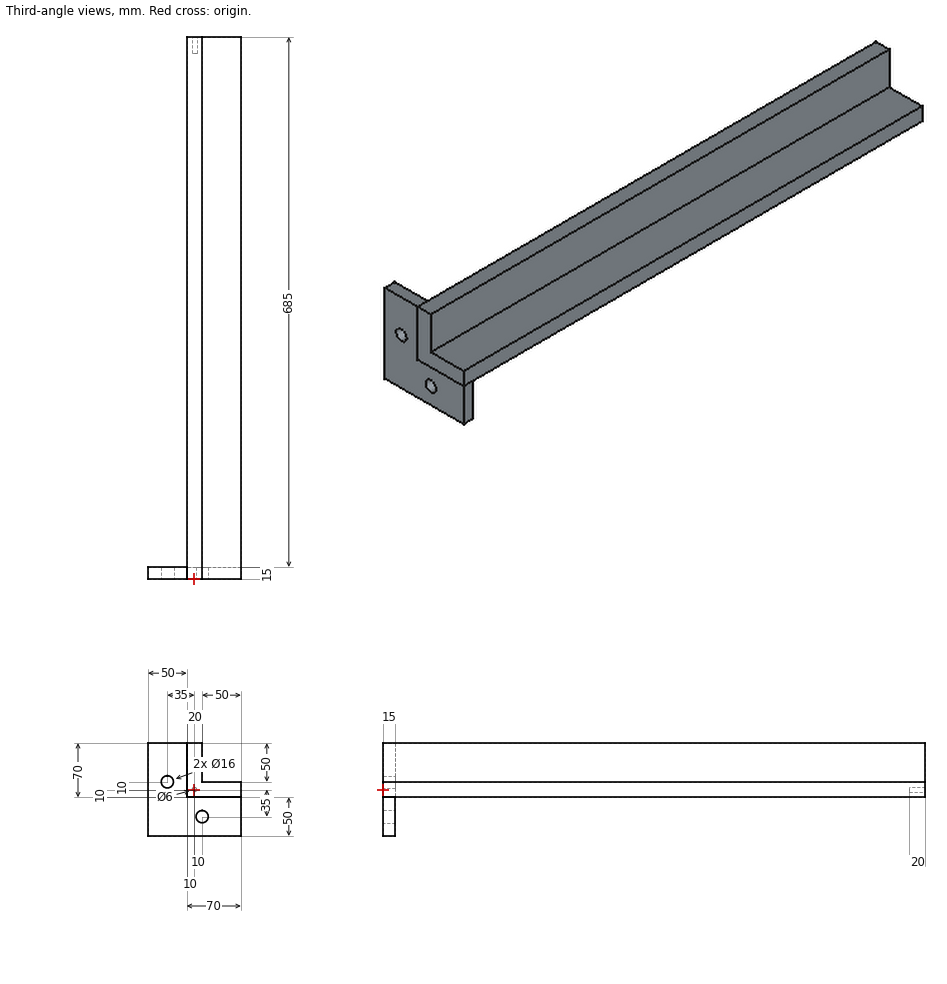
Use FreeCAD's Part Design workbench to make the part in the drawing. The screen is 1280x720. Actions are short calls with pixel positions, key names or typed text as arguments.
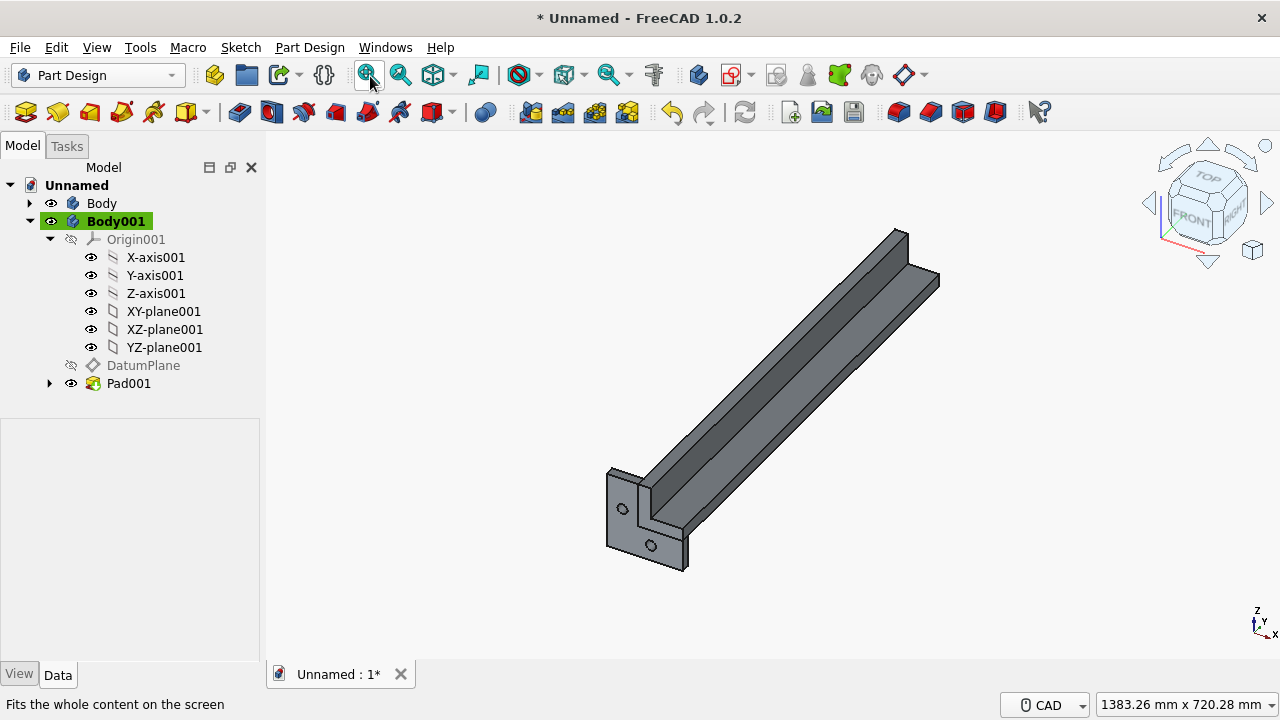
key(4)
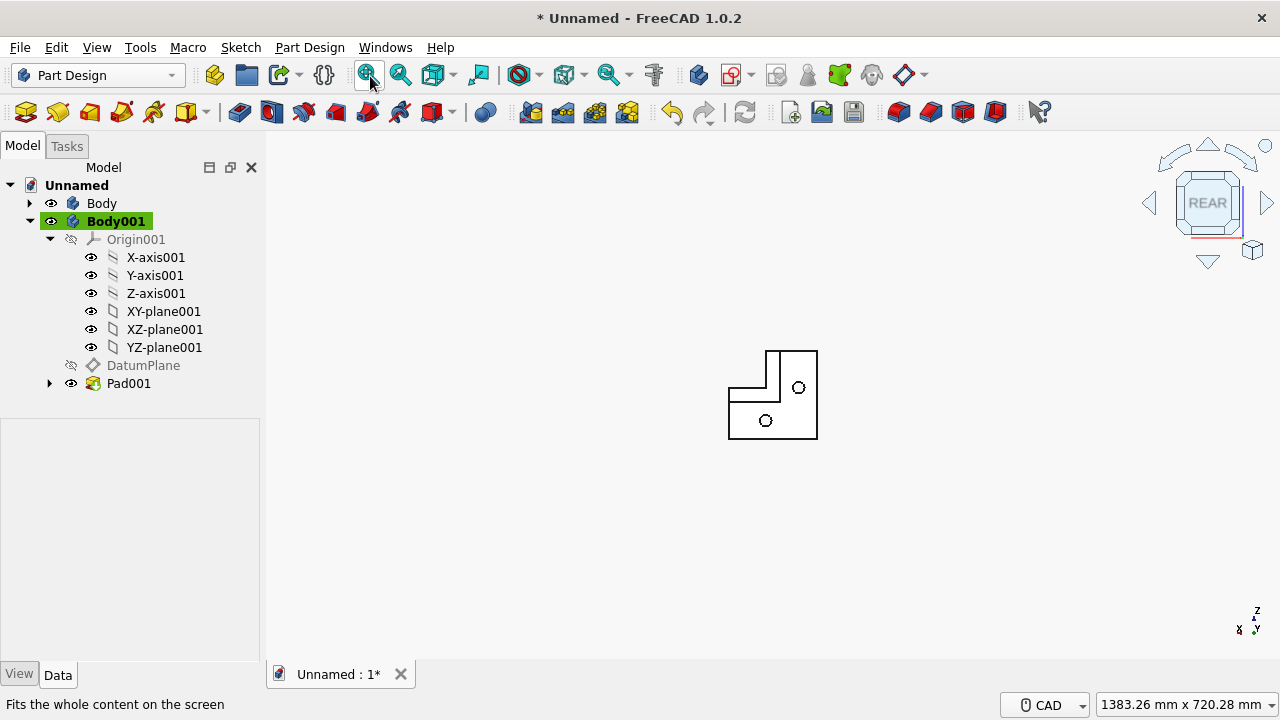
click(370, 76)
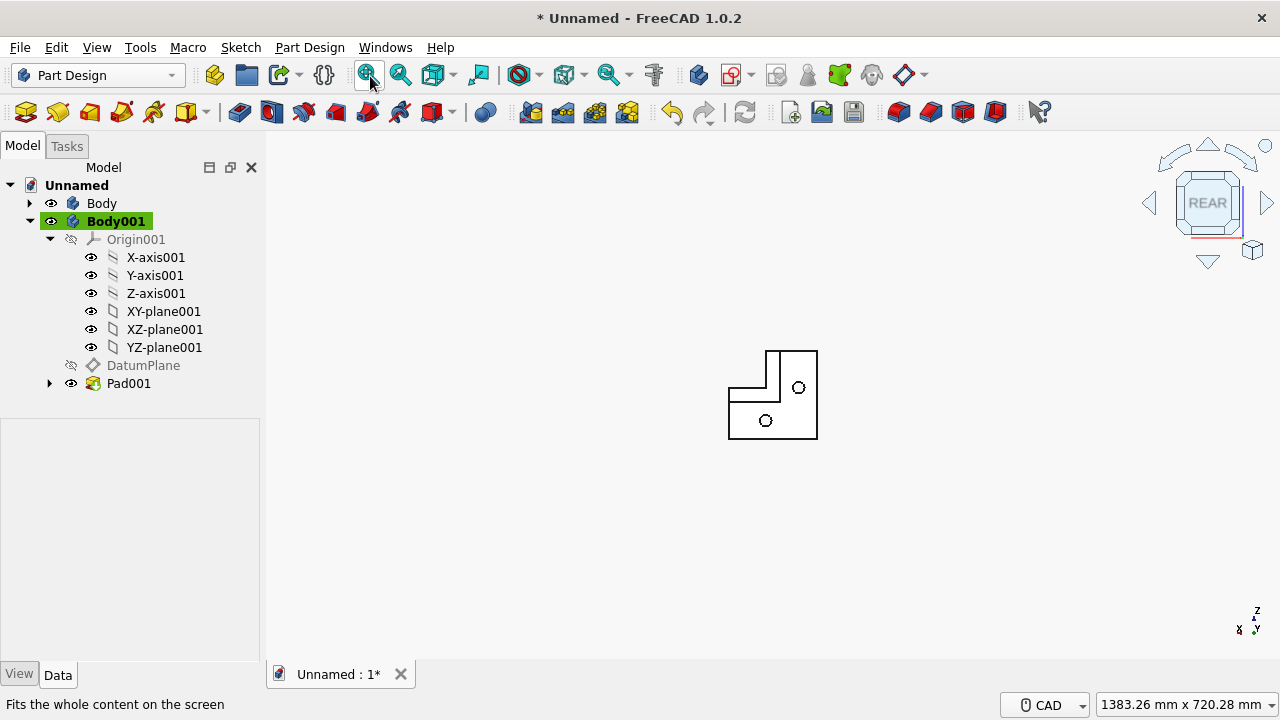
click(769, 390)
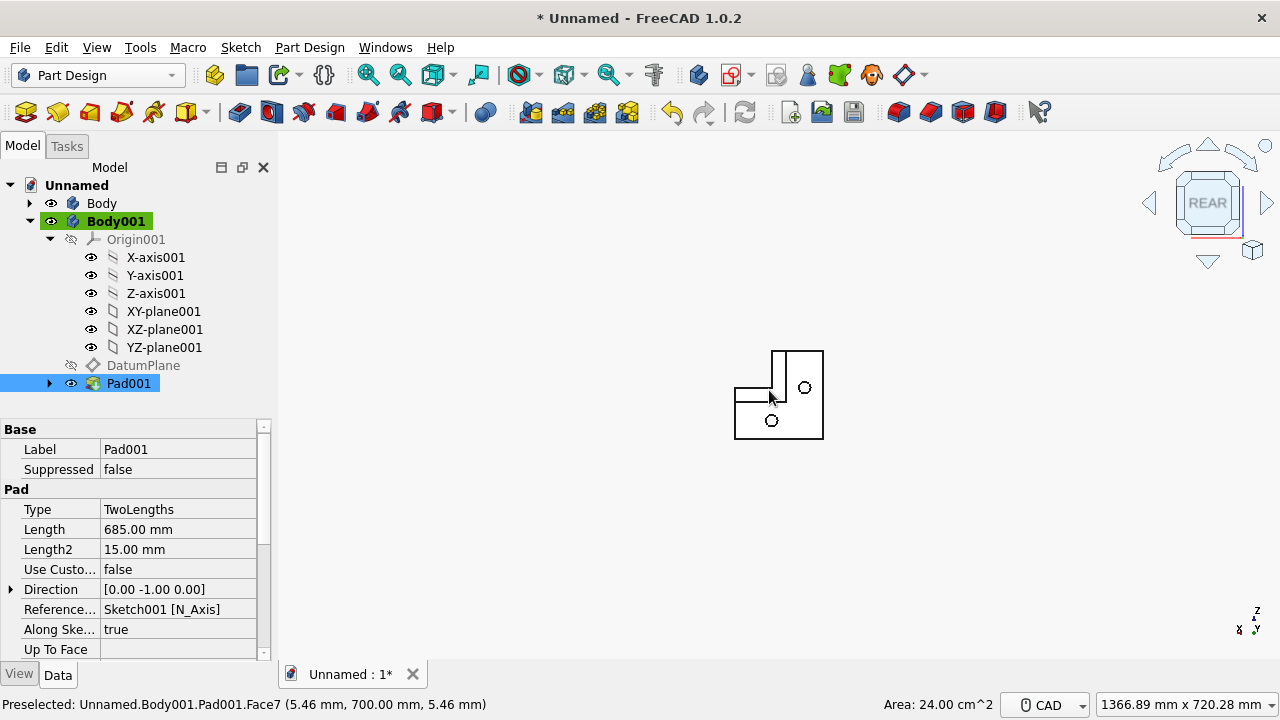
click(732, 76)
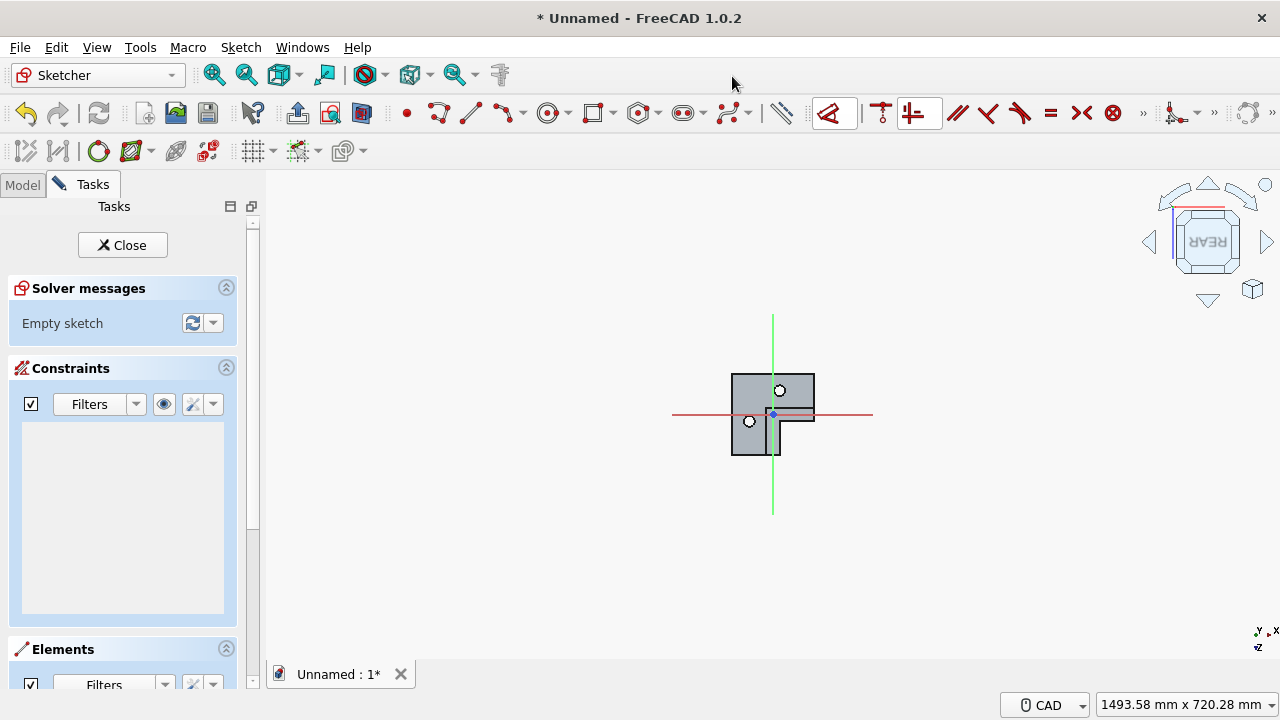
scroll(777, 414, up, 15)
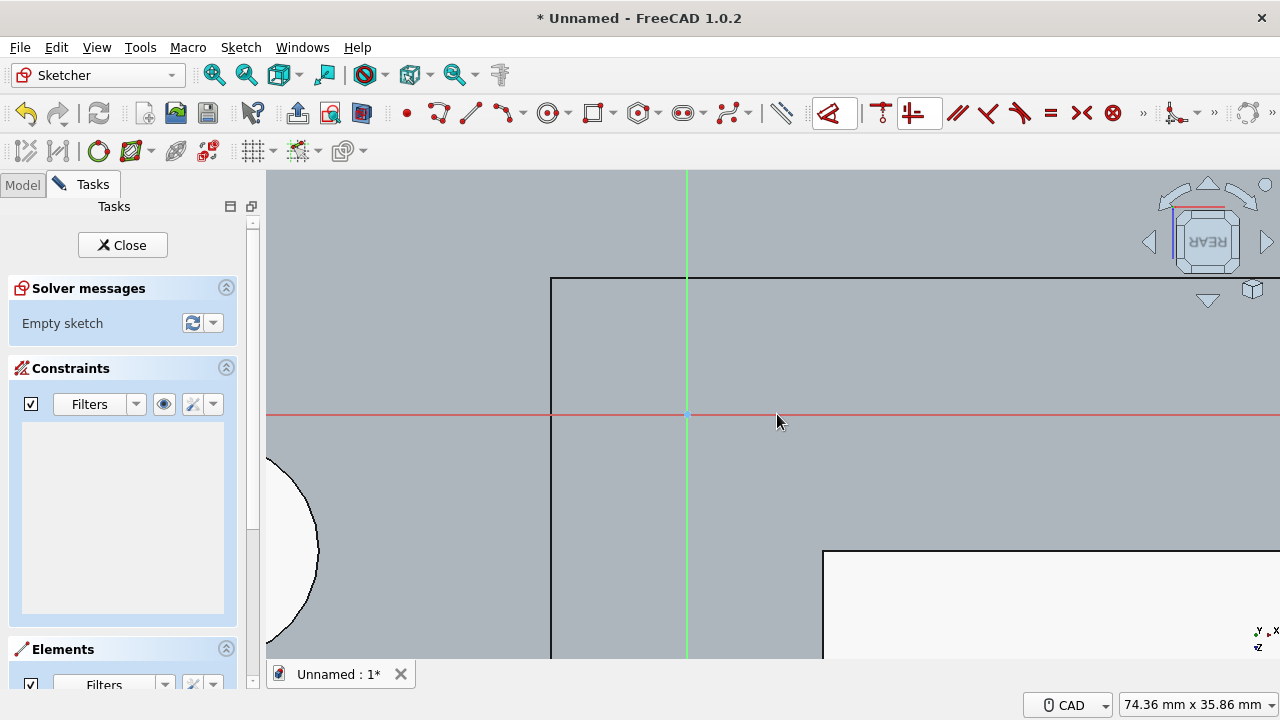
scroll(681, 414, up, 7)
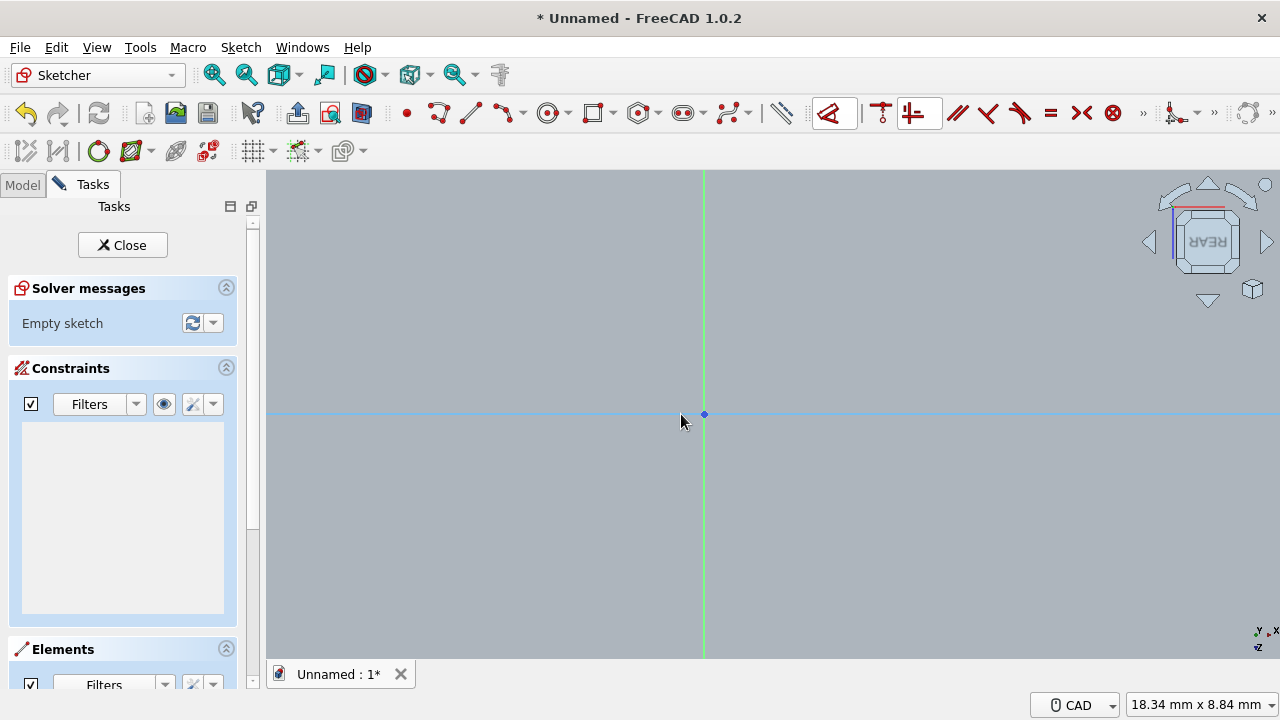
click(548, 114)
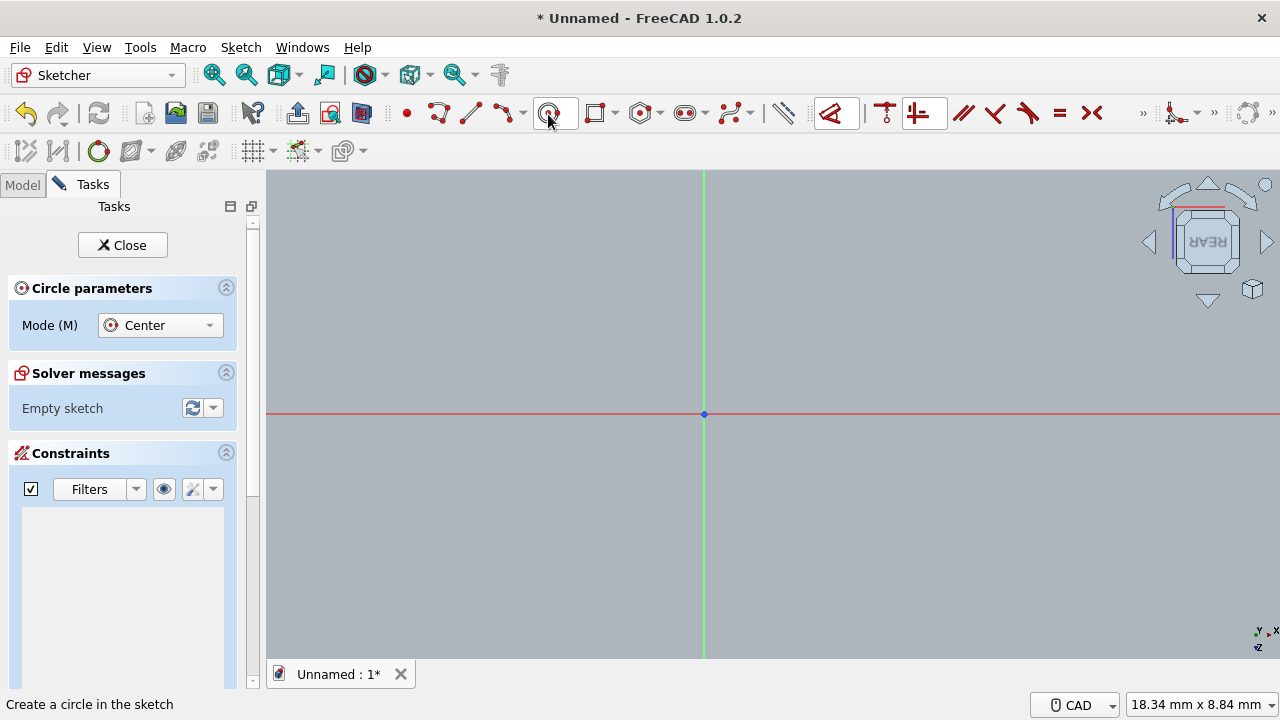
click(704, 414)
move(822, 297)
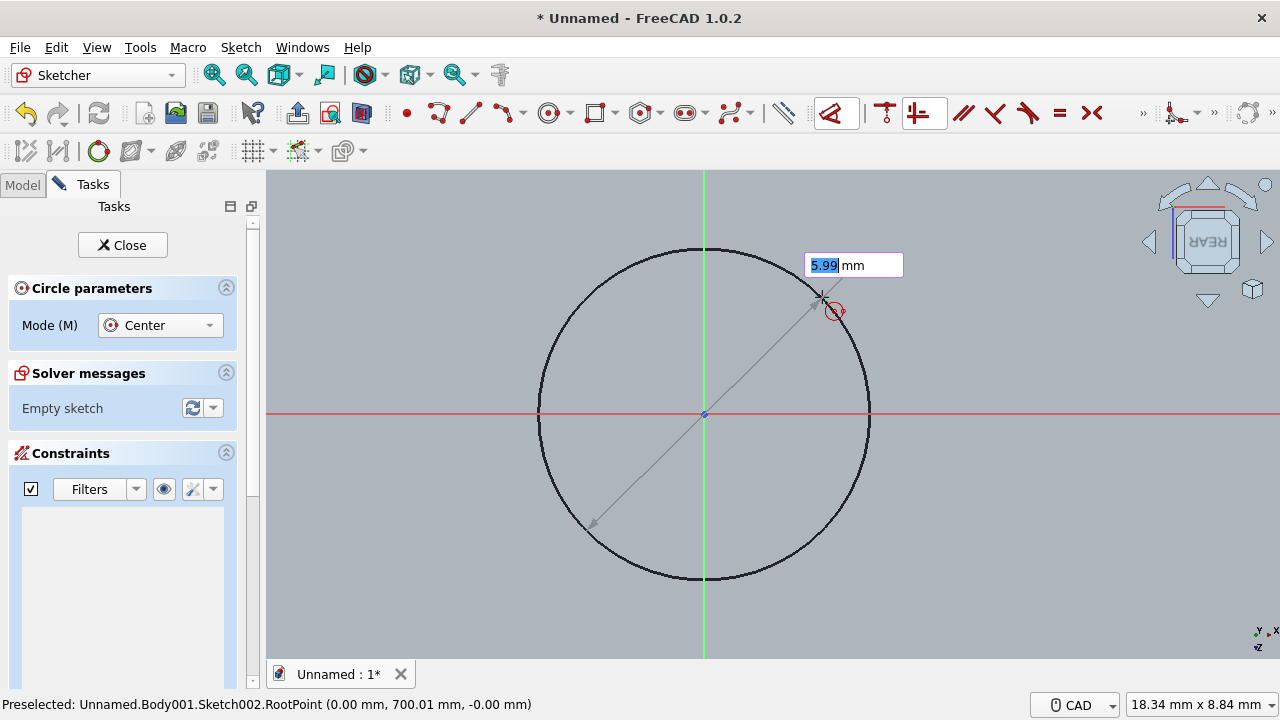
text(6)
key(Return)
key(Escape)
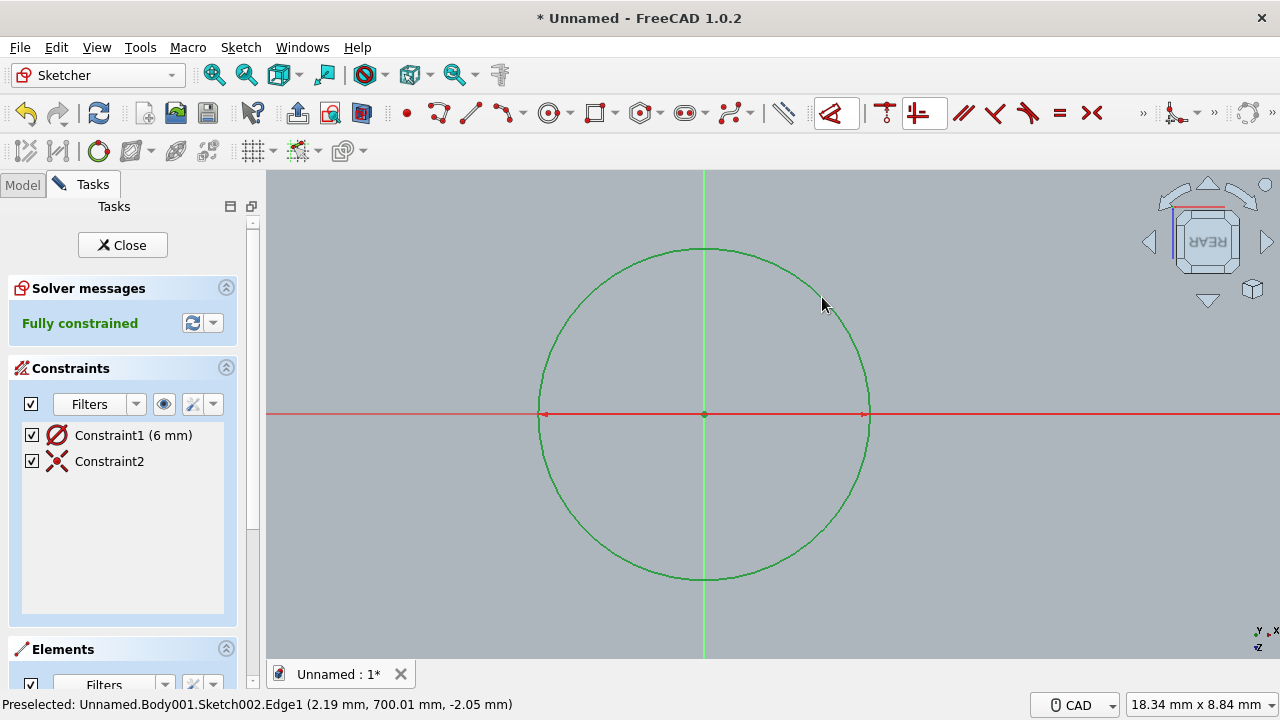
click(123, 245)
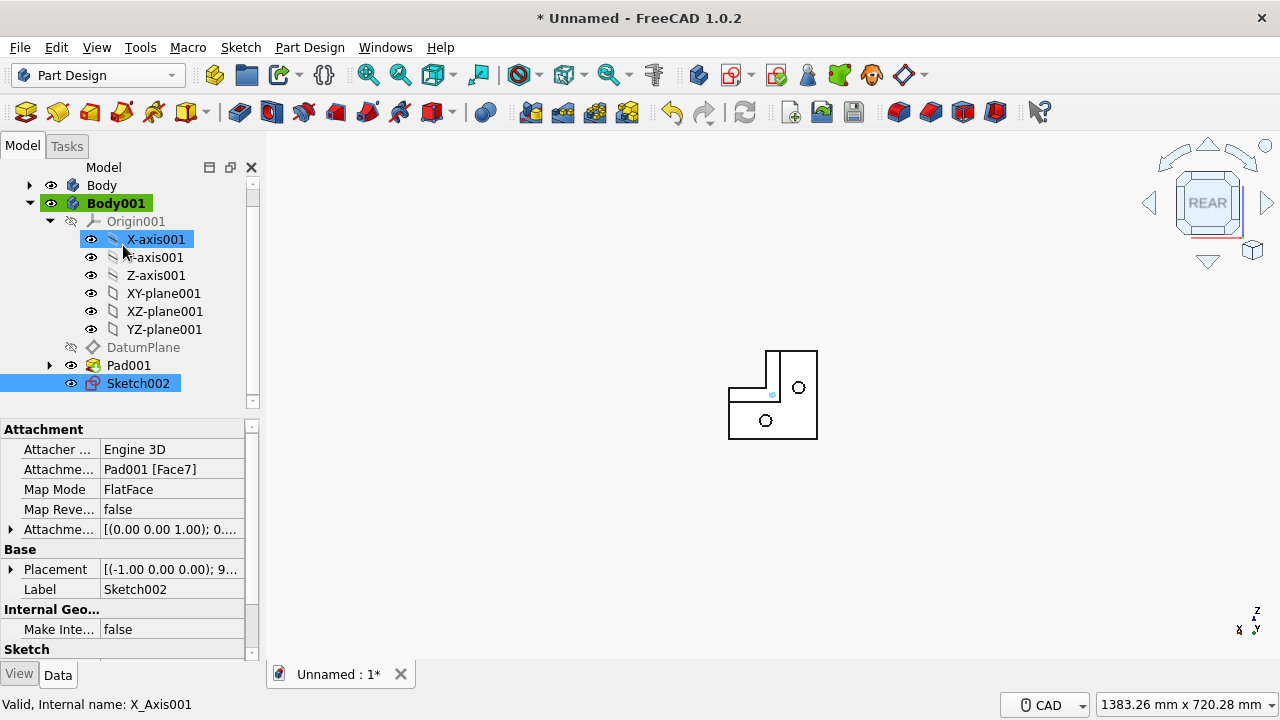
click(240, 112)